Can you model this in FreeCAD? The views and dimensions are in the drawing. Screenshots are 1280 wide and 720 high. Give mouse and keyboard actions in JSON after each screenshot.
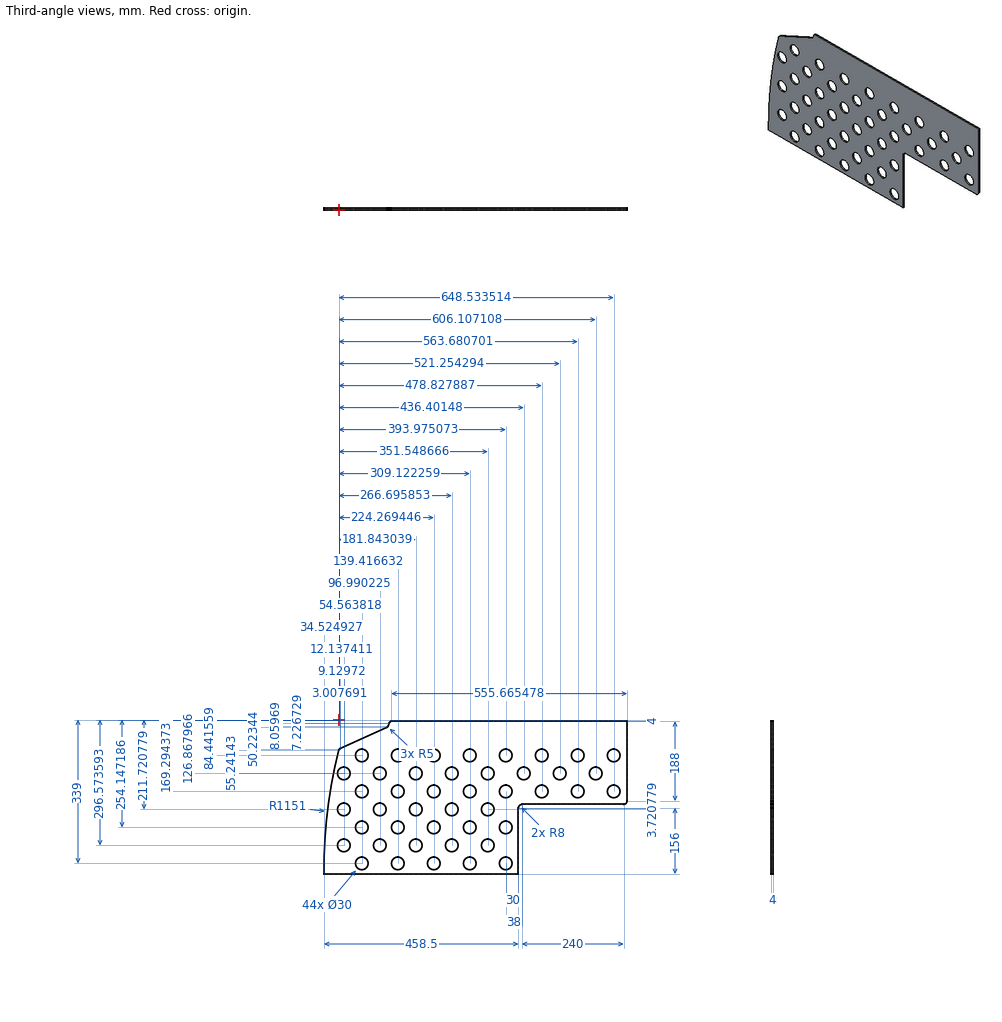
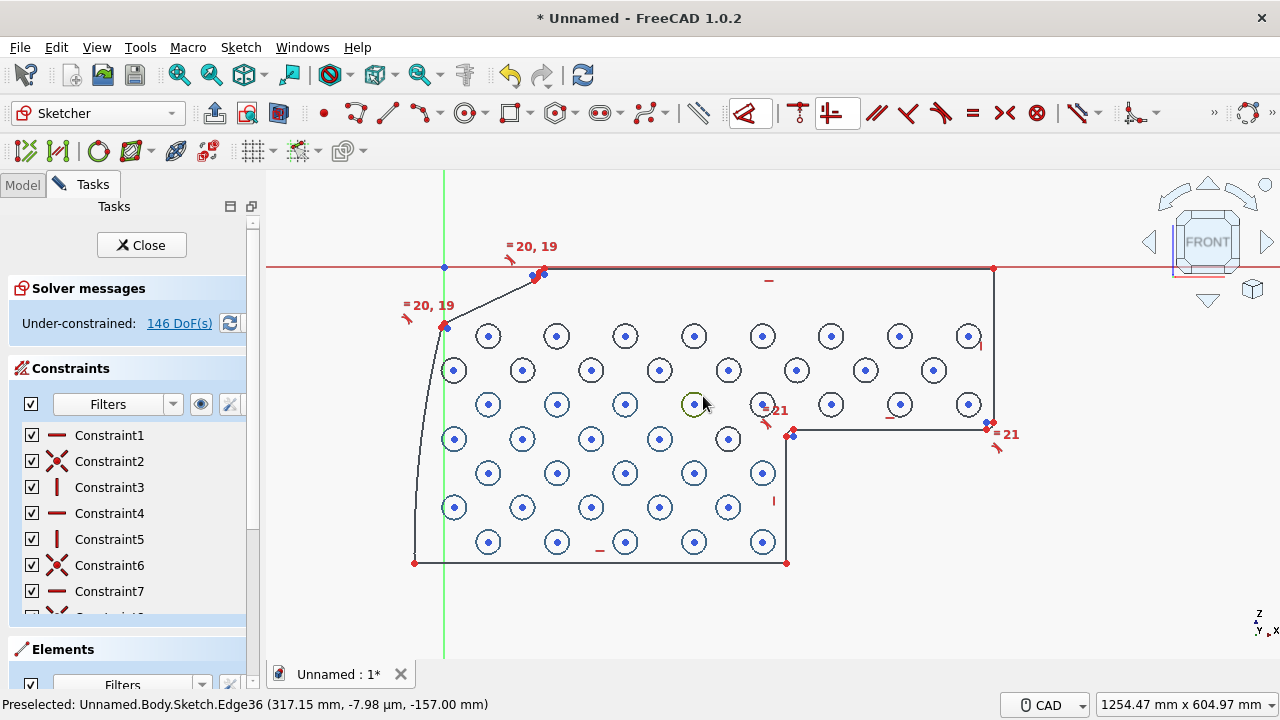
{"action": "left_click", "coordinate": [463, 362]}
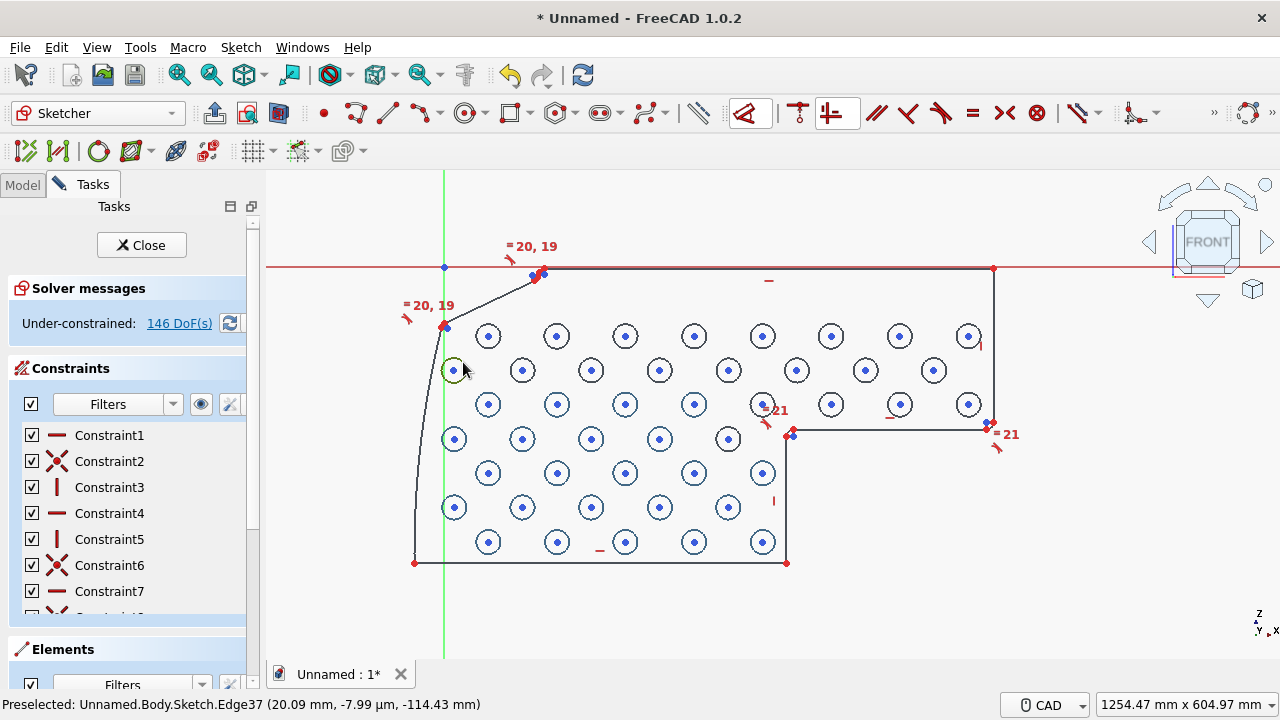
{"action": "left_click", "coordinate": [531, 362]}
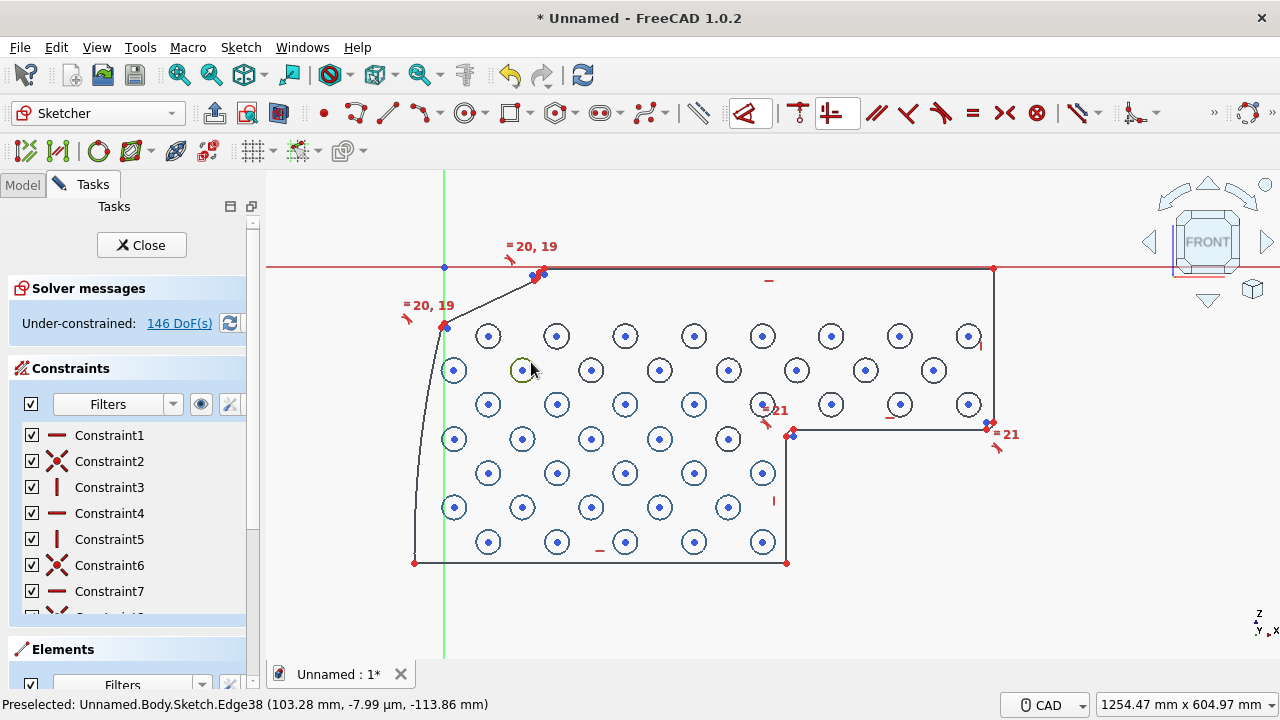
{"action": "left_click", "coordinate": [497, 328]}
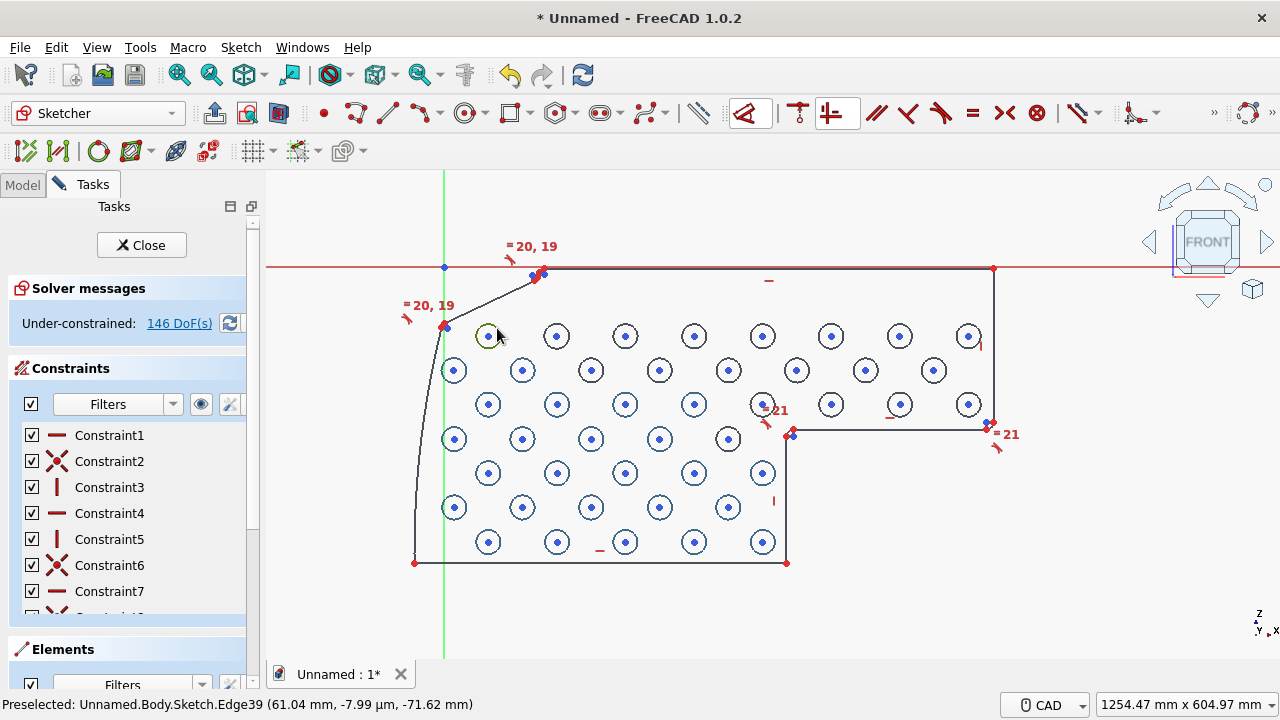
{"action": "left_click", "coordinate": [565, 327]}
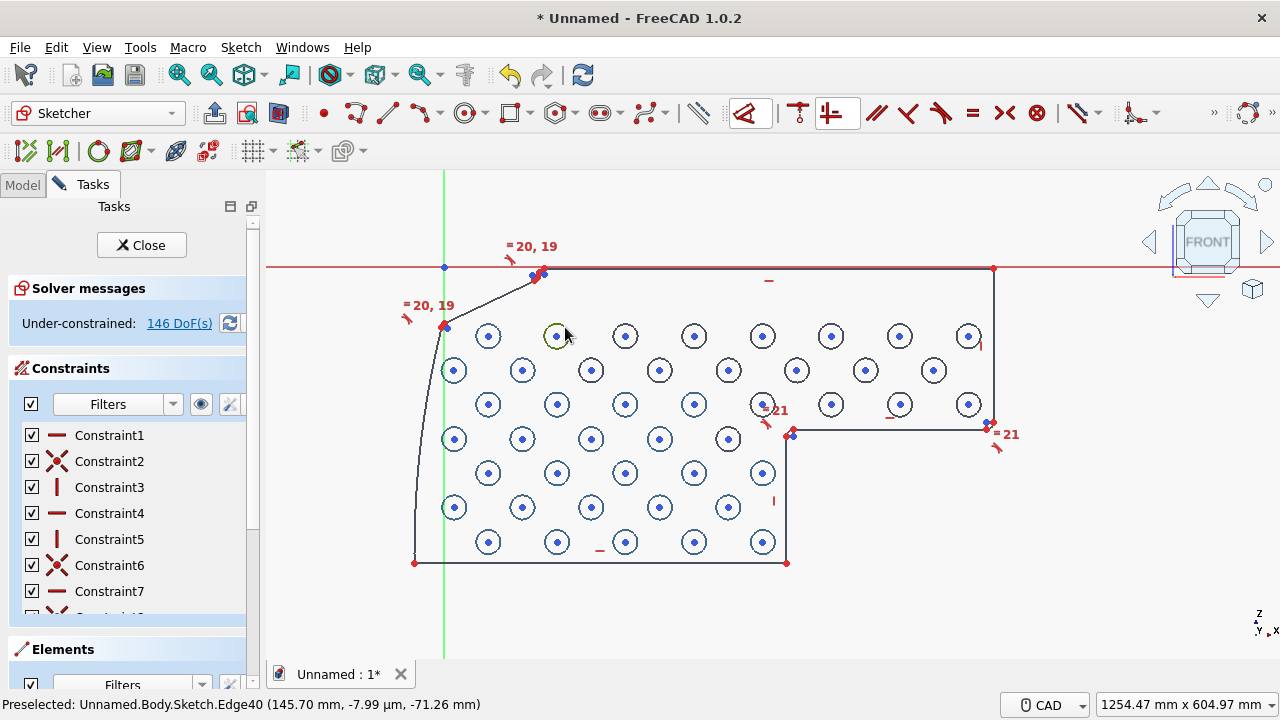
{"action": "left_click", "coordinate": [600, 362]}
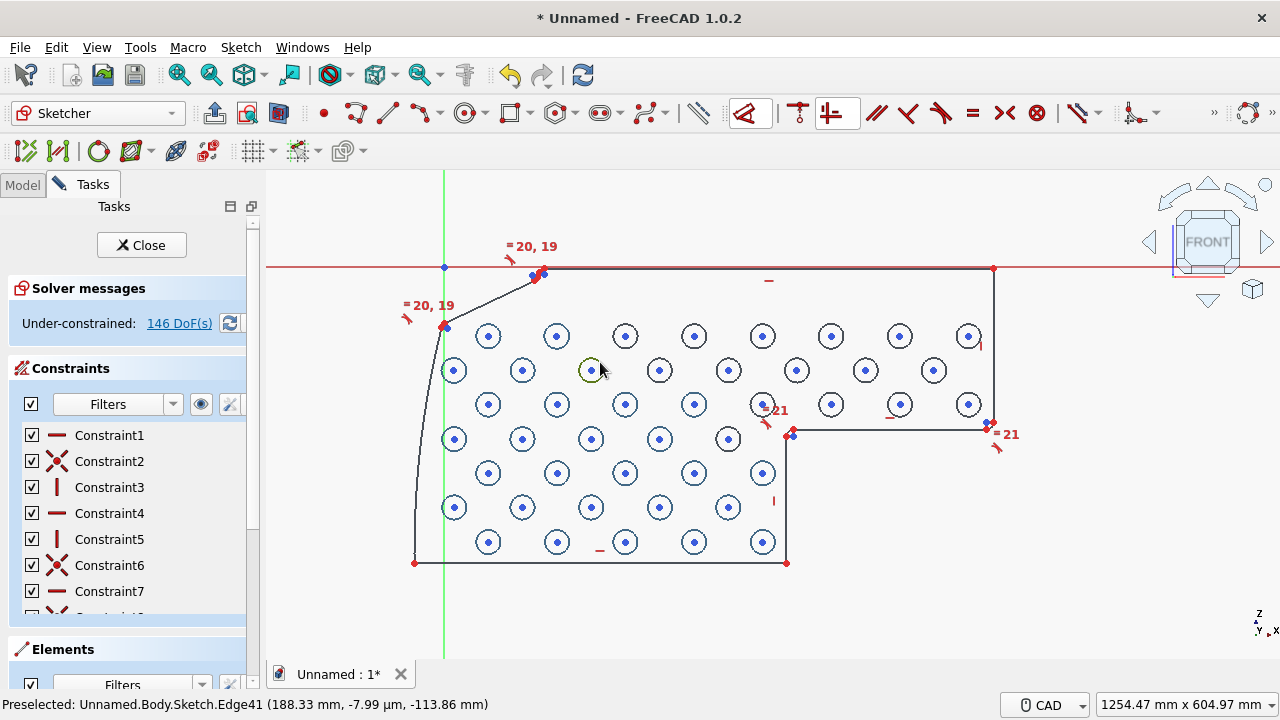
{"action": "left_click", "coordinate": [668, 362]}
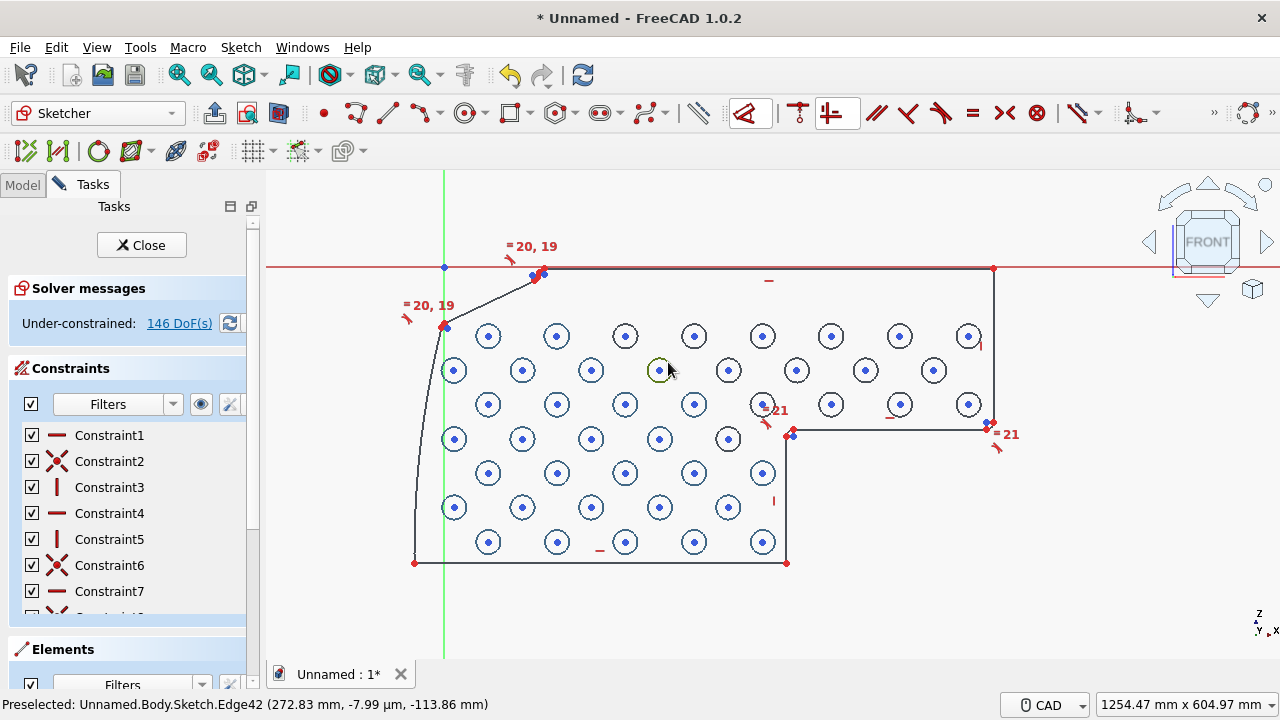
{"action": "left_click", "coordinate": [634, 328]}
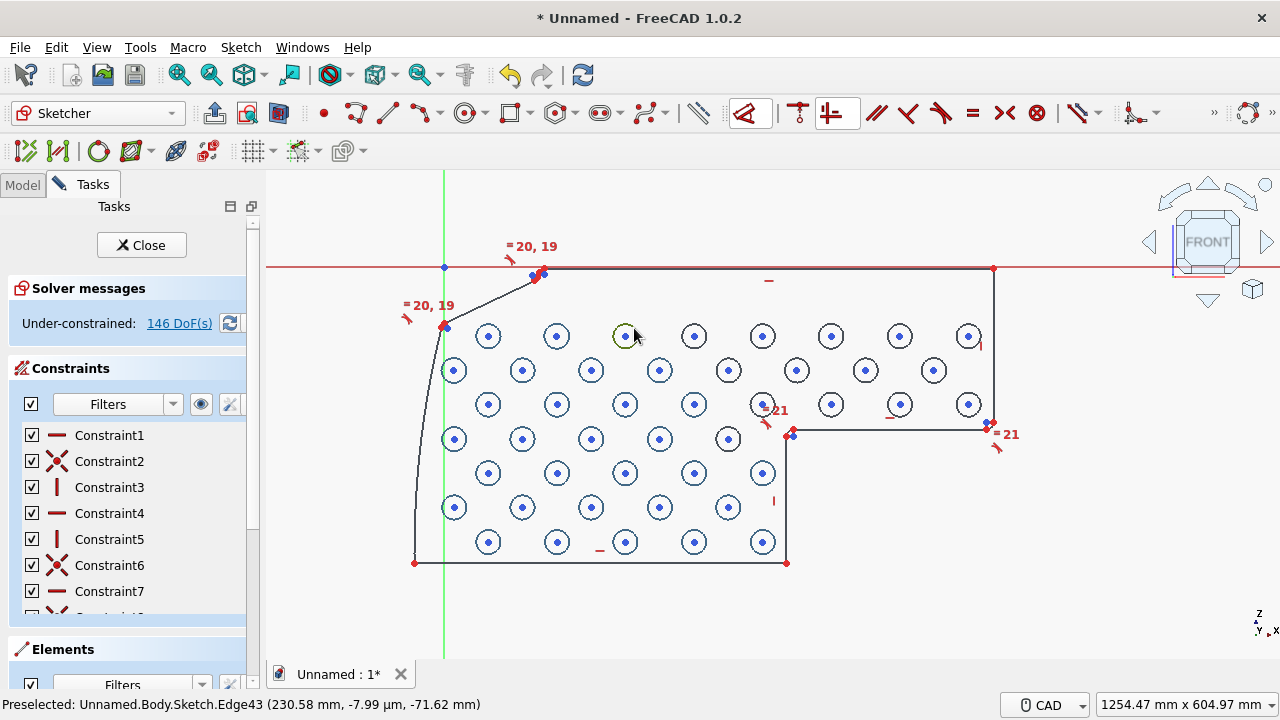
{"action": "left_click", "coordinate": [703, 328]}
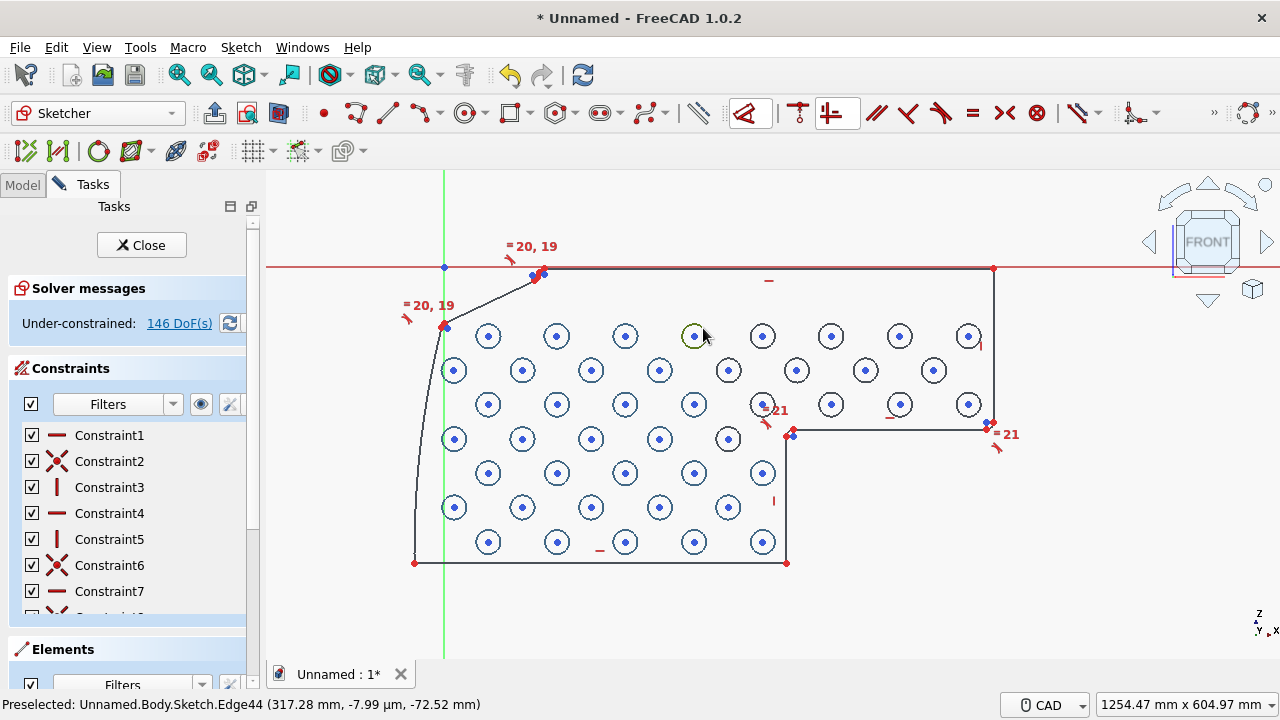
{"action": "left_click", "coordinate": [737, 431]}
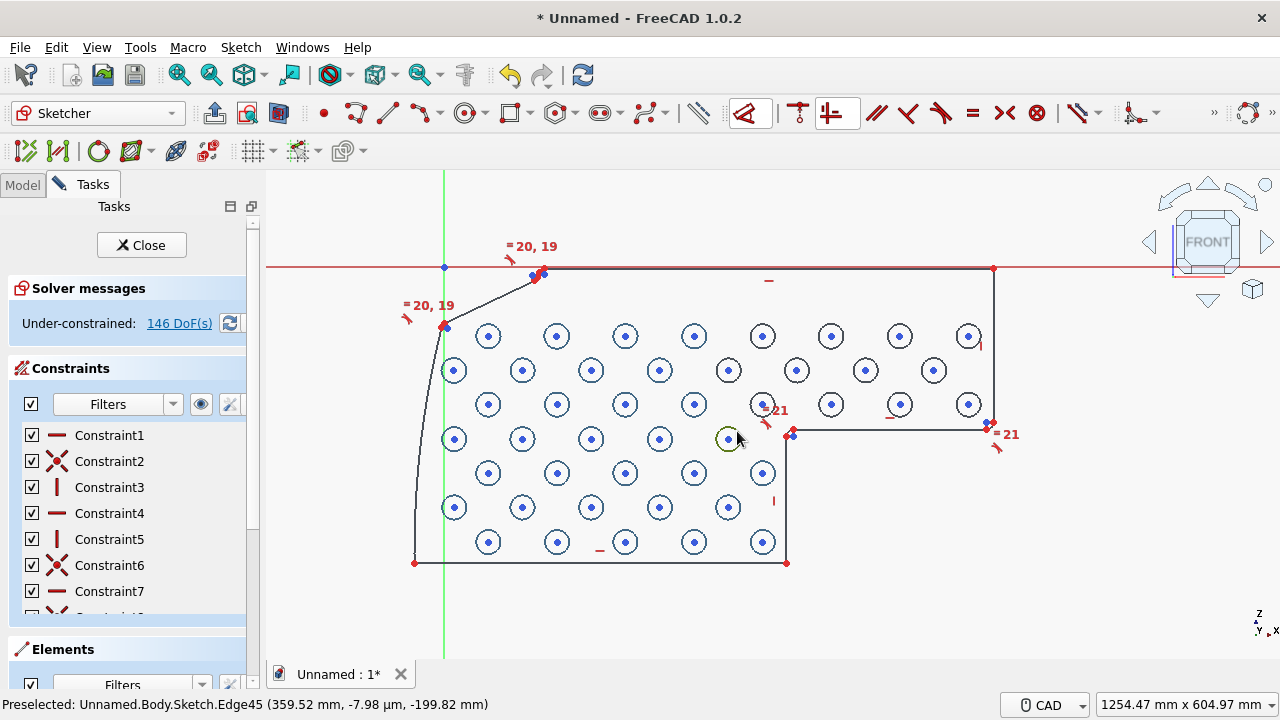
{"action": "left_click", "coordinate": [771, 396]}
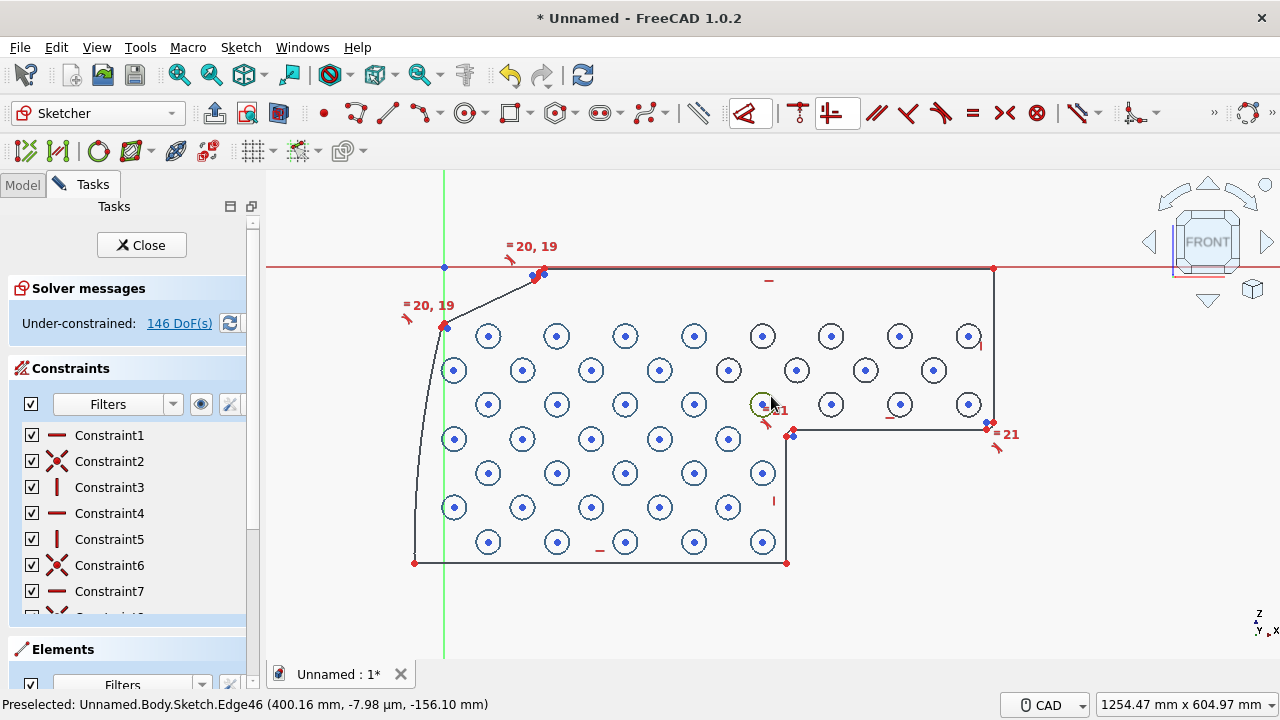
{"action": "left_click", "coordinate": [840, 396]}